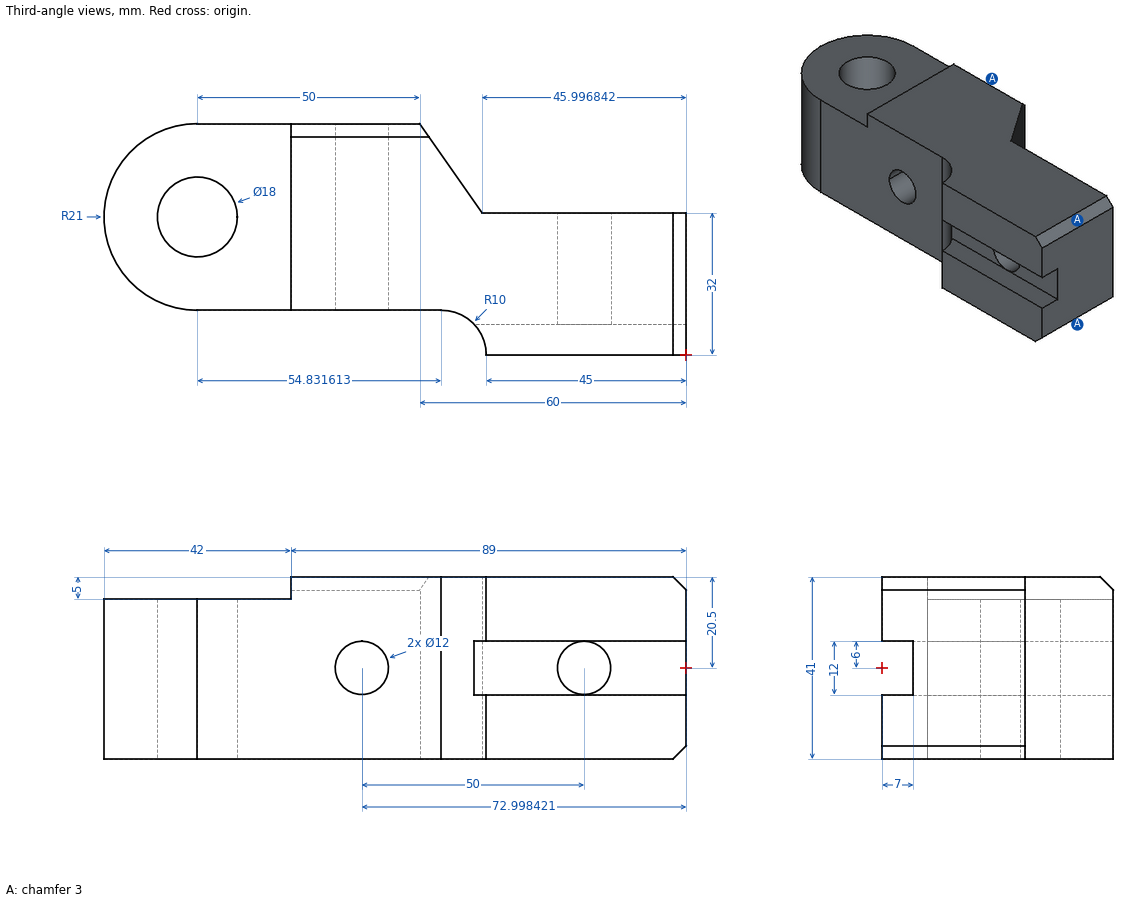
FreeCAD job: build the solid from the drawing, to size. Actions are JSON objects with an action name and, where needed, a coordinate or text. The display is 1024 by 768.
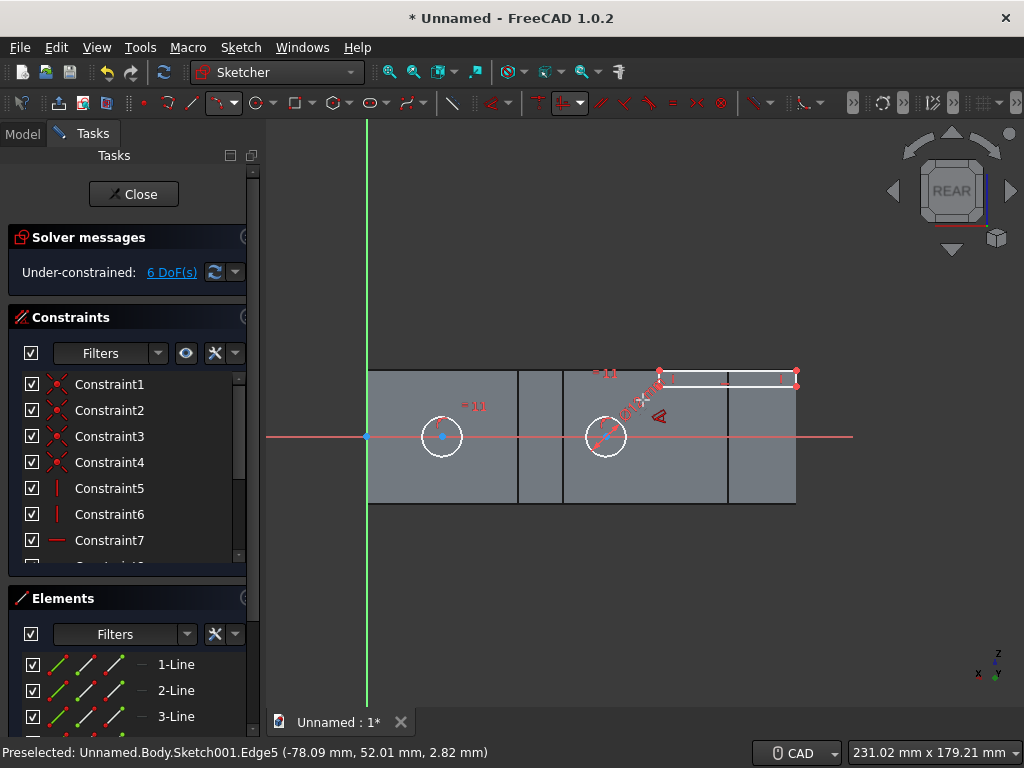
{"action": "scroll", "coordinate": [659, 379], "scroll_direction": "up", "scroll_amount": 5}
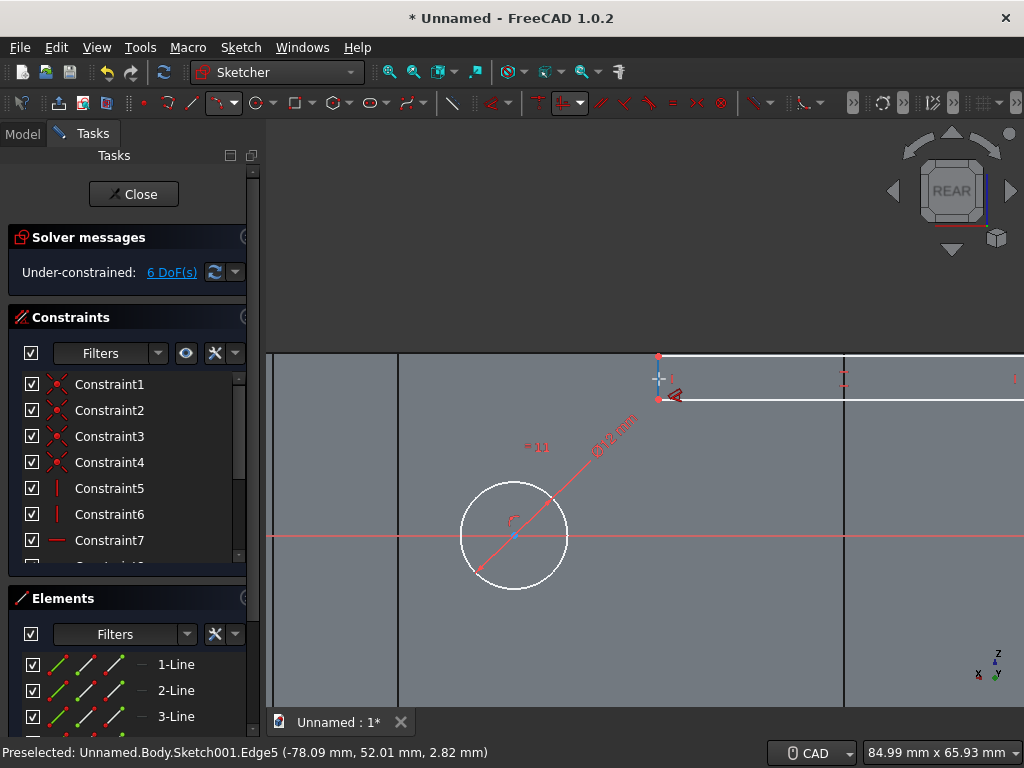
{"action": "left_click", "coordinate": [658, 378]}
{"action": "left_click", "coordinate": [692, 378]}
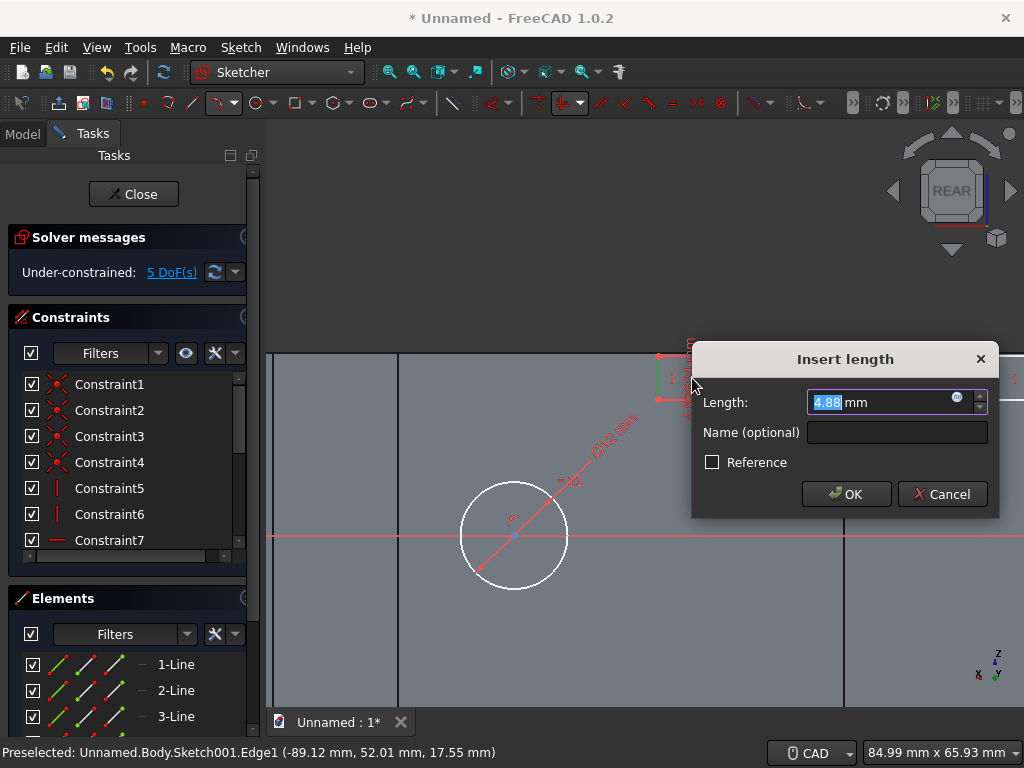
{"action": "type", "text": "5"}
{"action": "key", "text": "Return"}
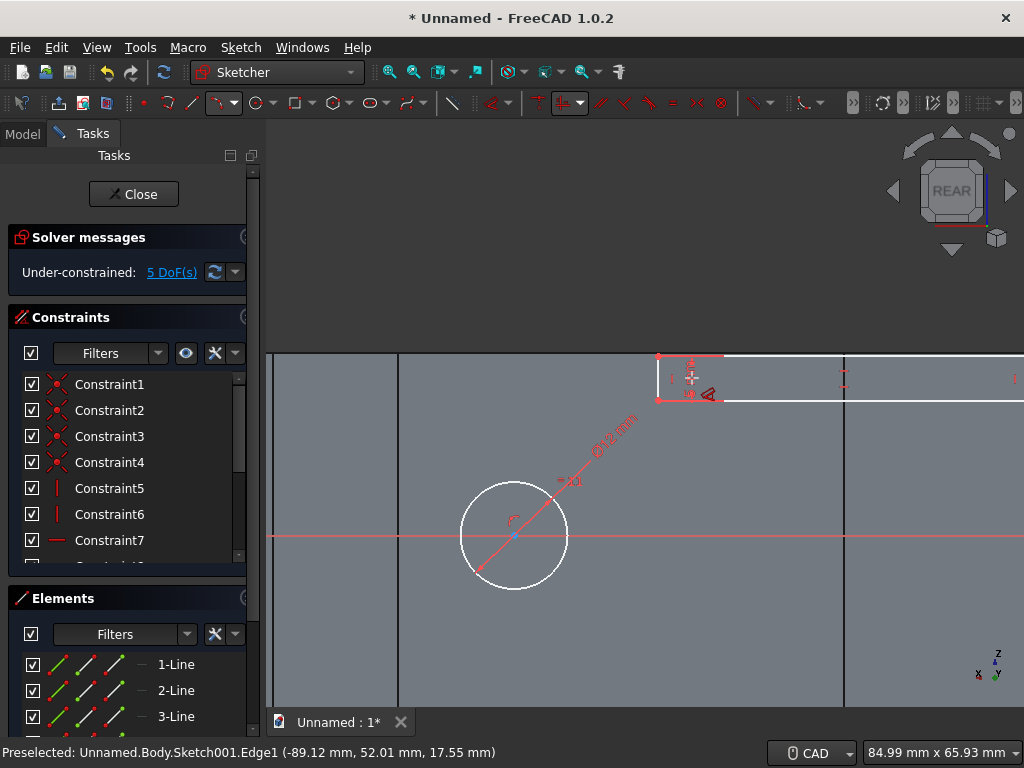
{"action": "left_click", "coordinate": [770, 401]}
{"action": "left_click", "coordinate": [759, 435]}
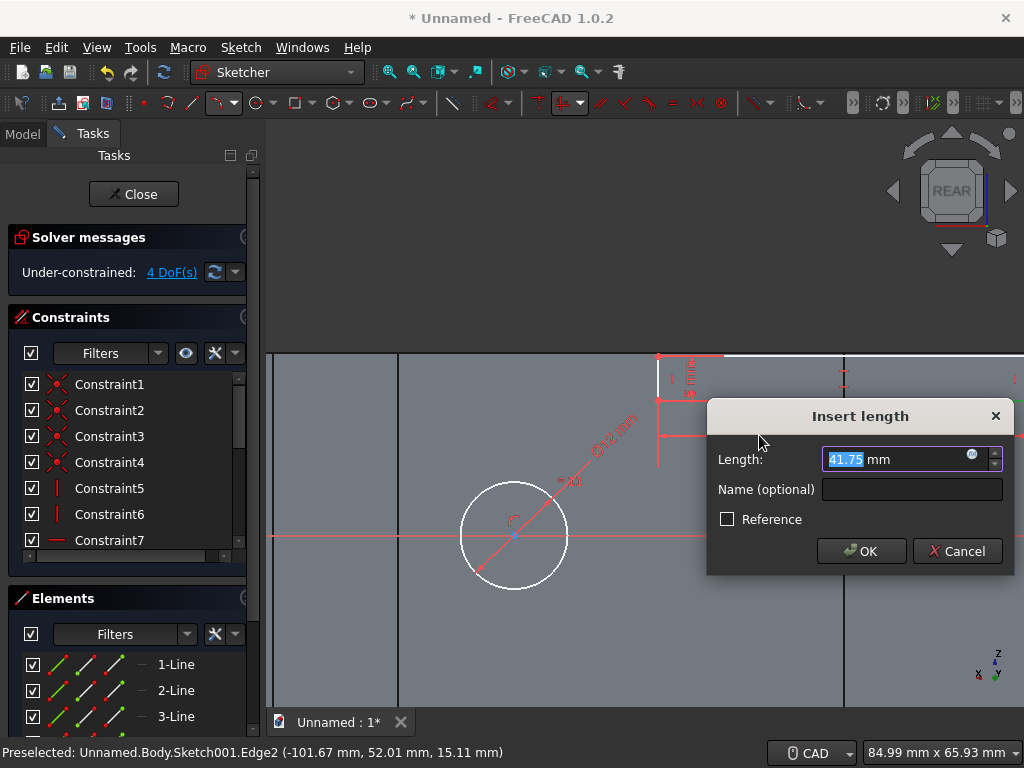
{"action": "type", "text": "42"}
{"action": "key", "text": "Return"}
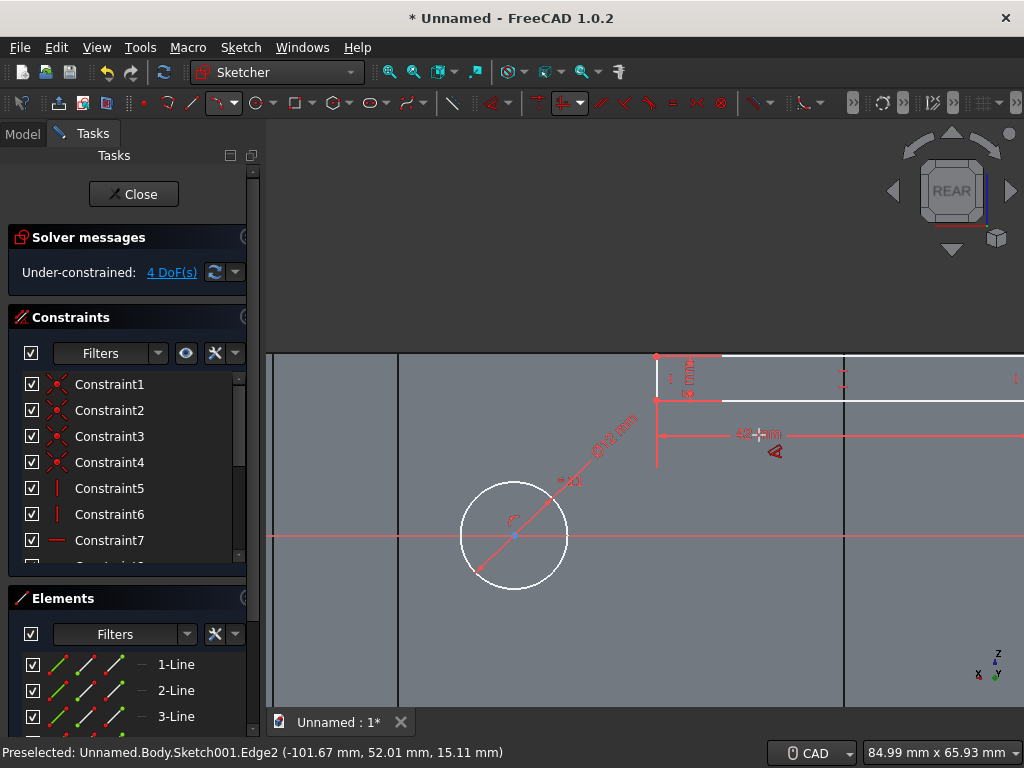
{"action": "left_click", "coordinate": [657, 356]}
{"action": "left_click", "coordinate": [475, 322]}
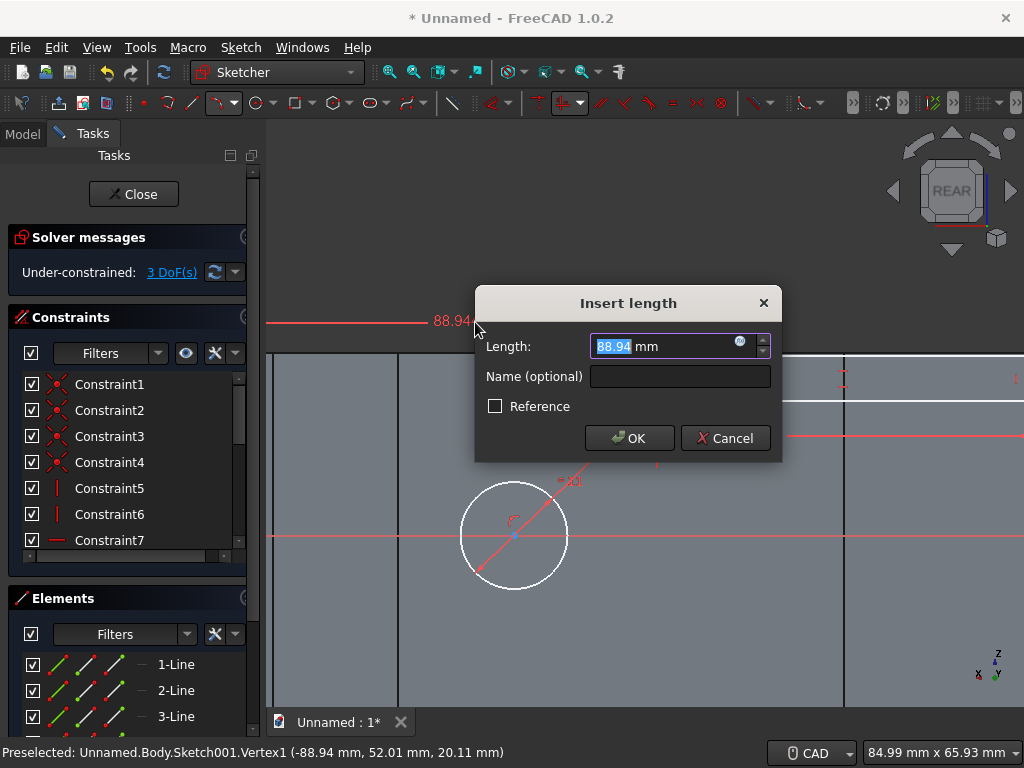
{"action": "type", "text": "89"}
{"action": "key", "text": "Return"}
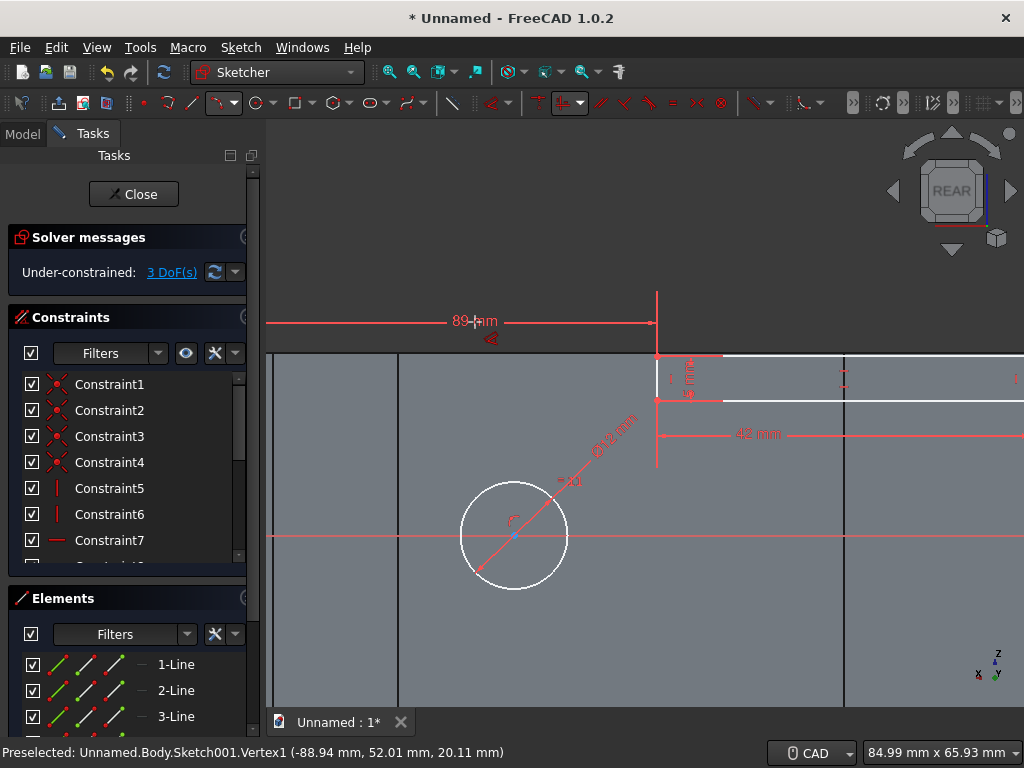
{"action": "left_click", "coordinate": [514, 536]}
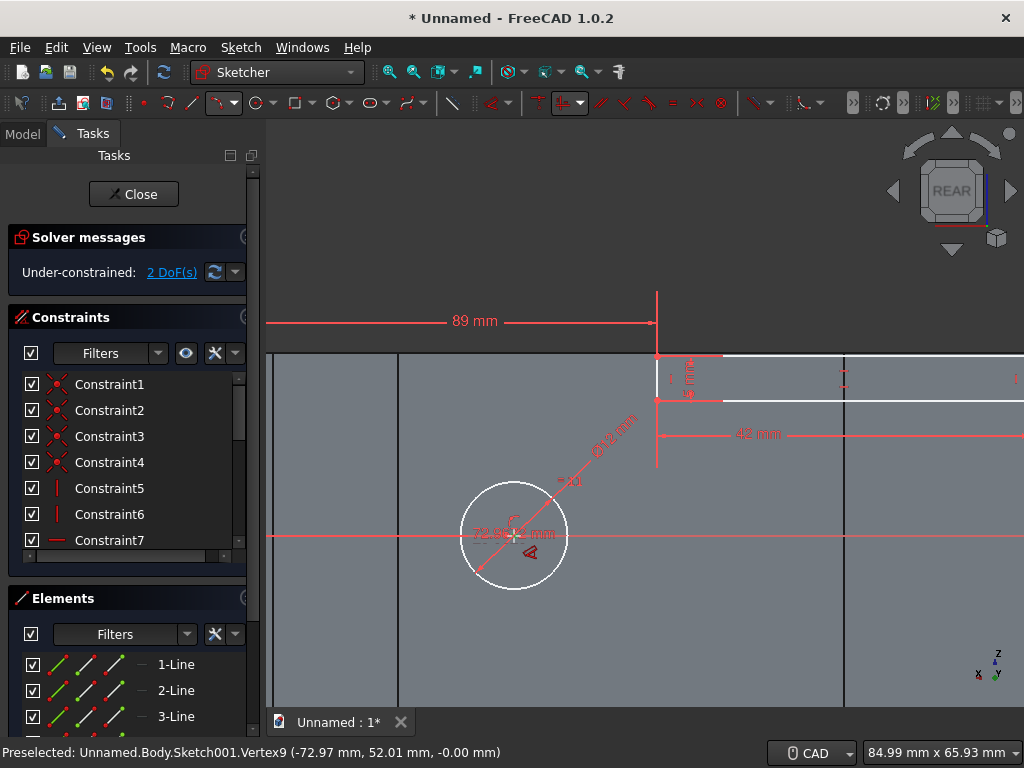
{"action": "scroll", "coordinate": [652, 379], "scroll_direction": "down", "scroll_amount": 5}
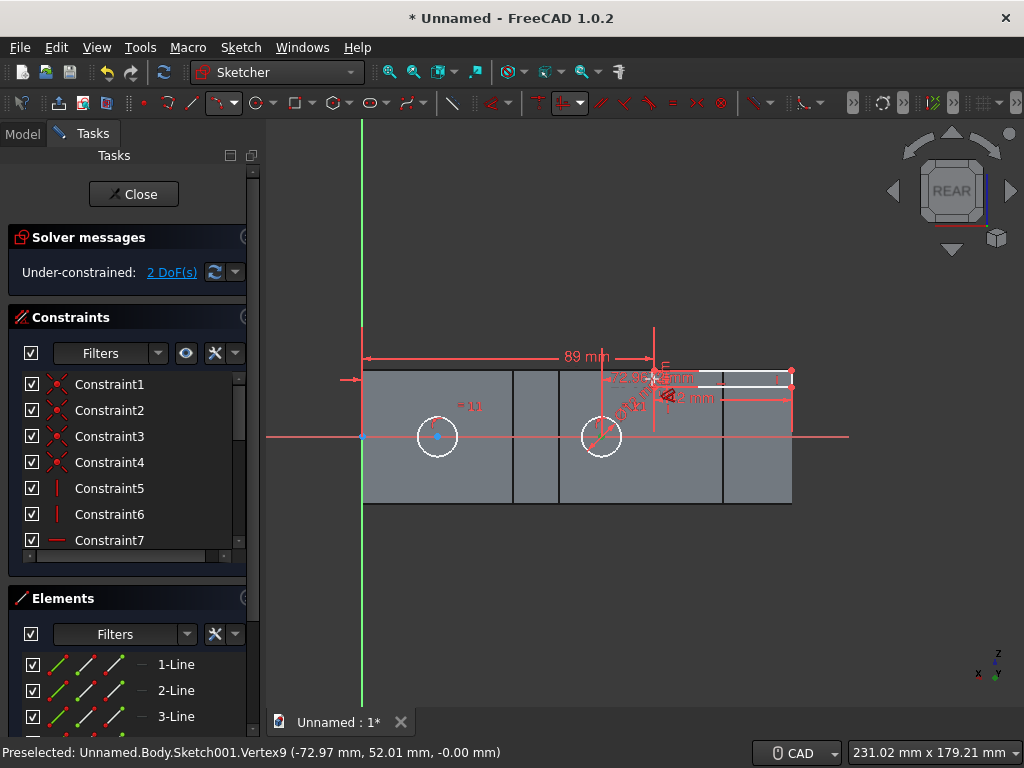
{"action": "left_click", "coordinate": [438, 437]}
{"action": "left_click", "coordinate": [520, 471]}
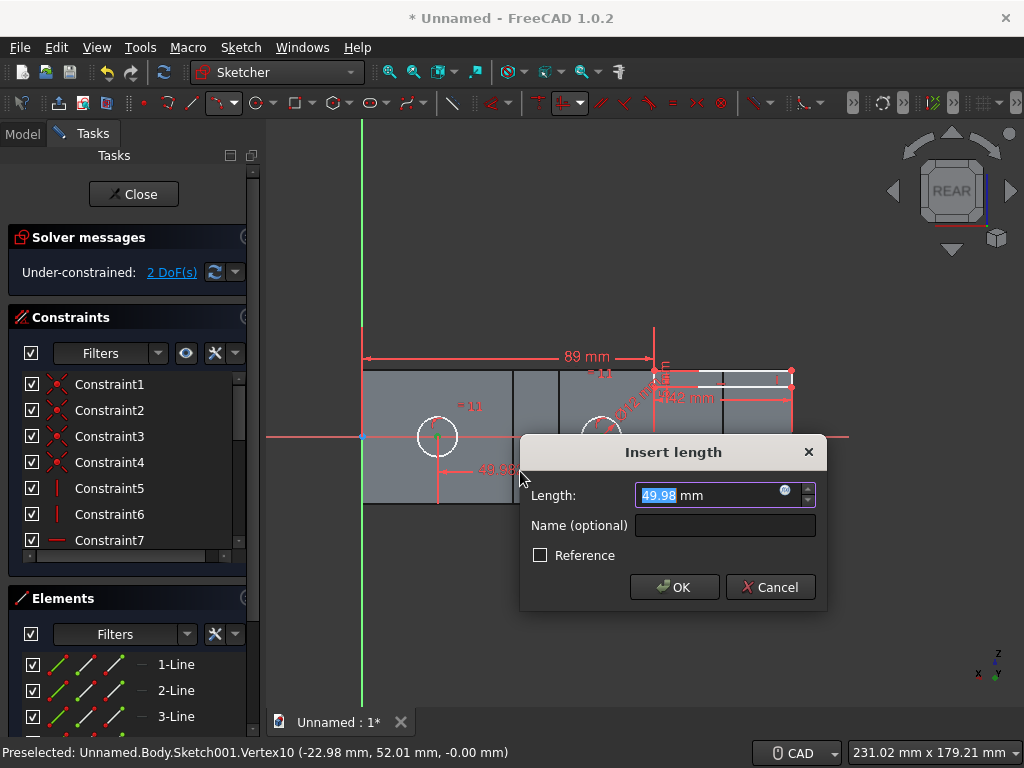
{"action": "type", "text": "50"}
{"action": "key", "text": "Return"}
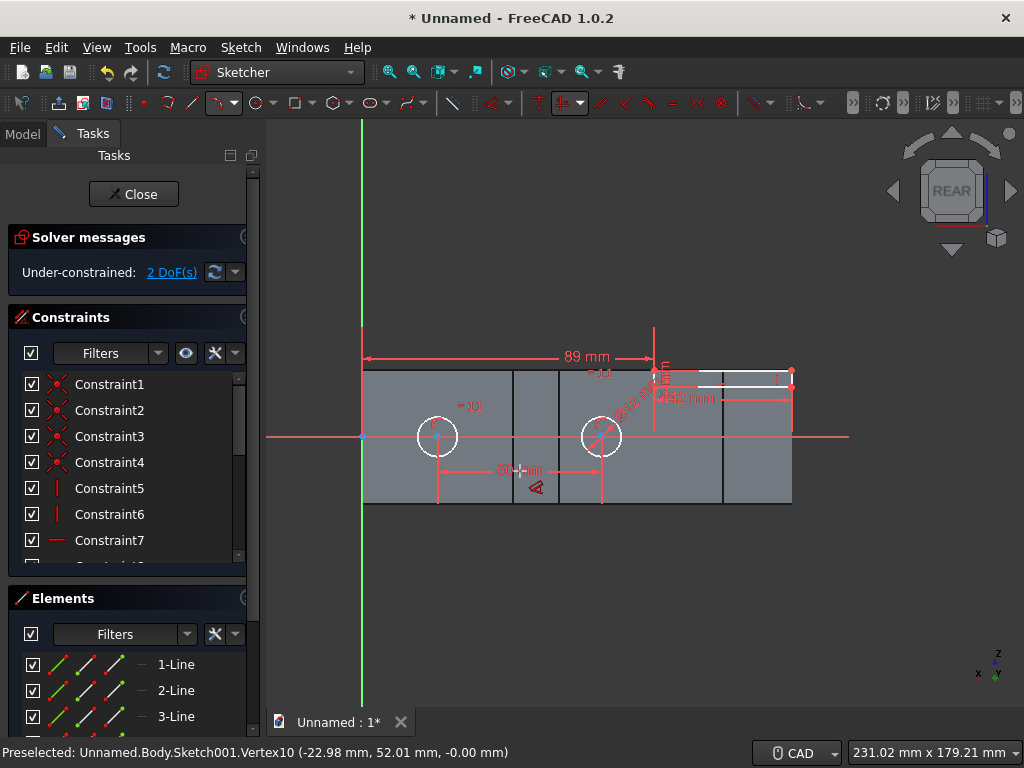
{"action": "left_click", "coordinate": [654, 371]}
{"action": "left_click", "coordinate": [328, 404]}